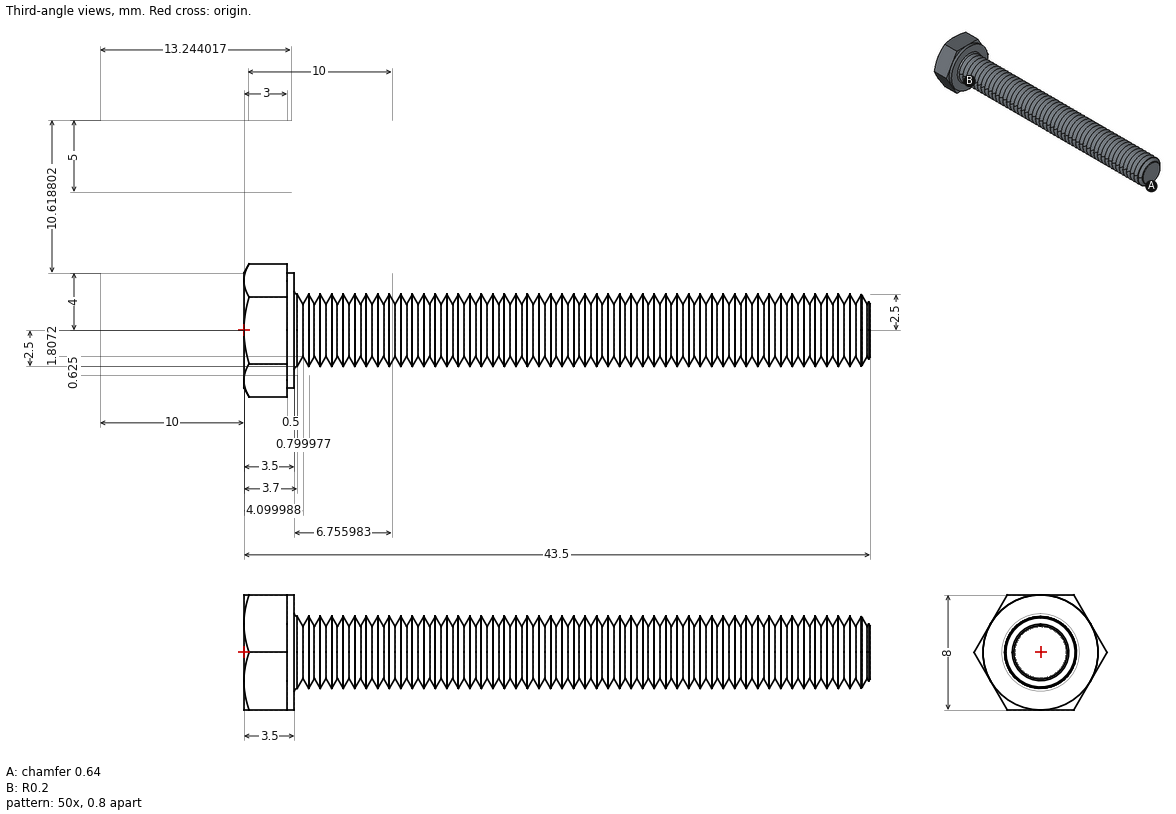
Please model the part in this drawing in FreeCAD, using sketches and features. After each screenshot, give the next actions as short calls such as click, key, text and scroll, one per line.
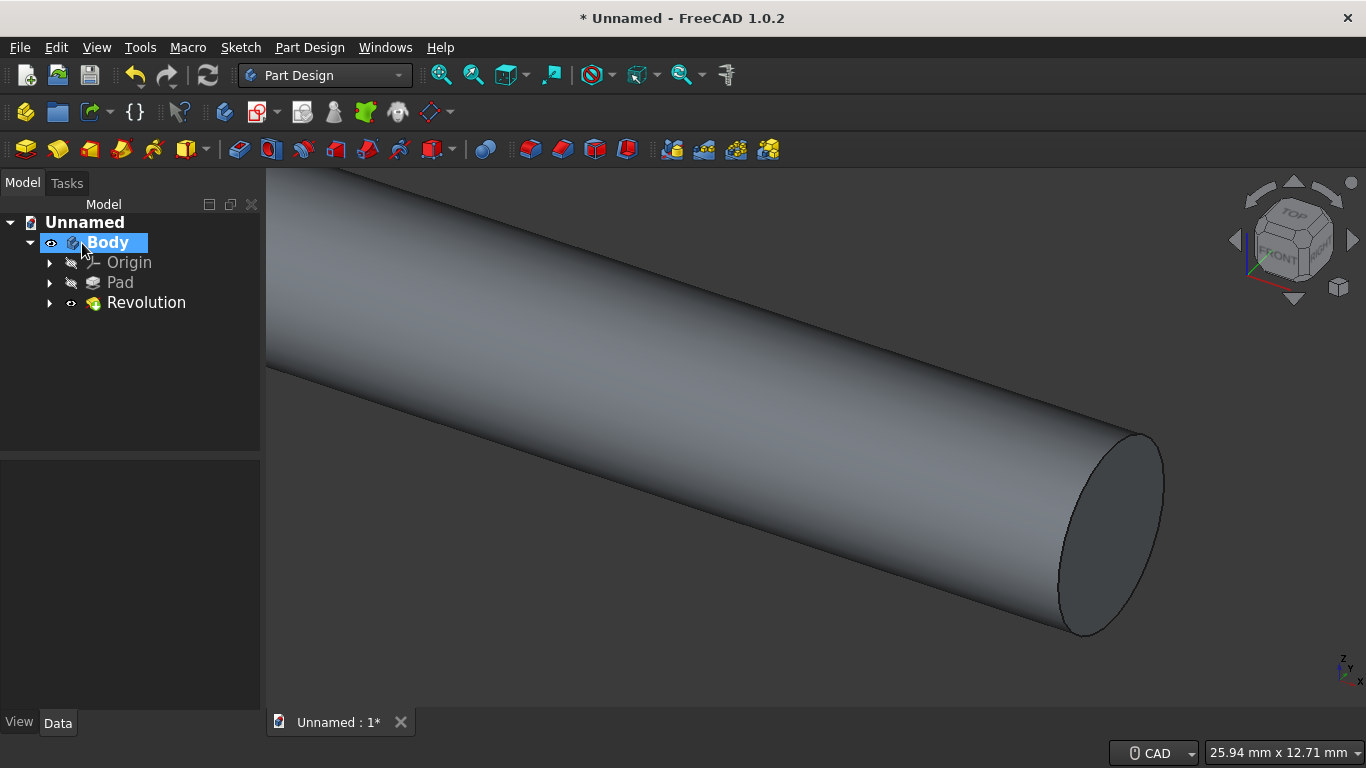
click(442, 76)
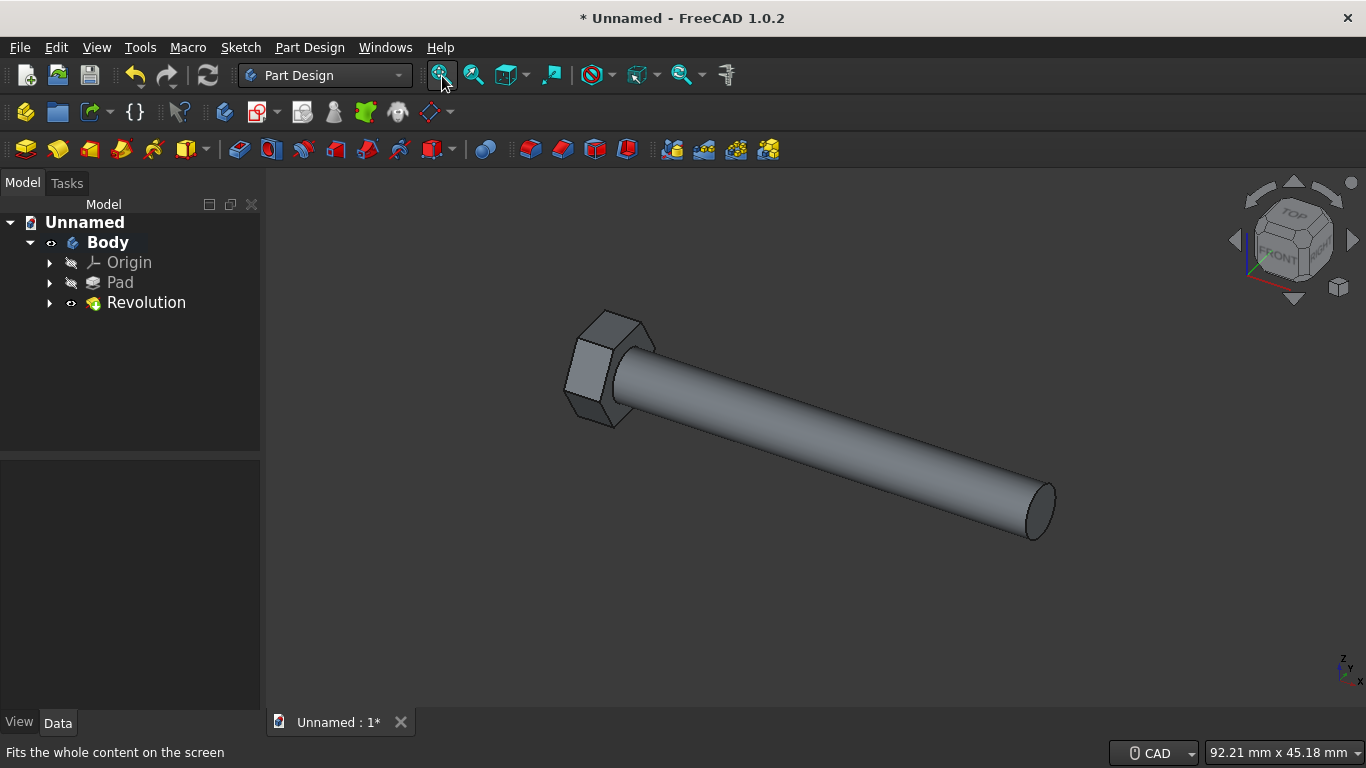
click(258, 112)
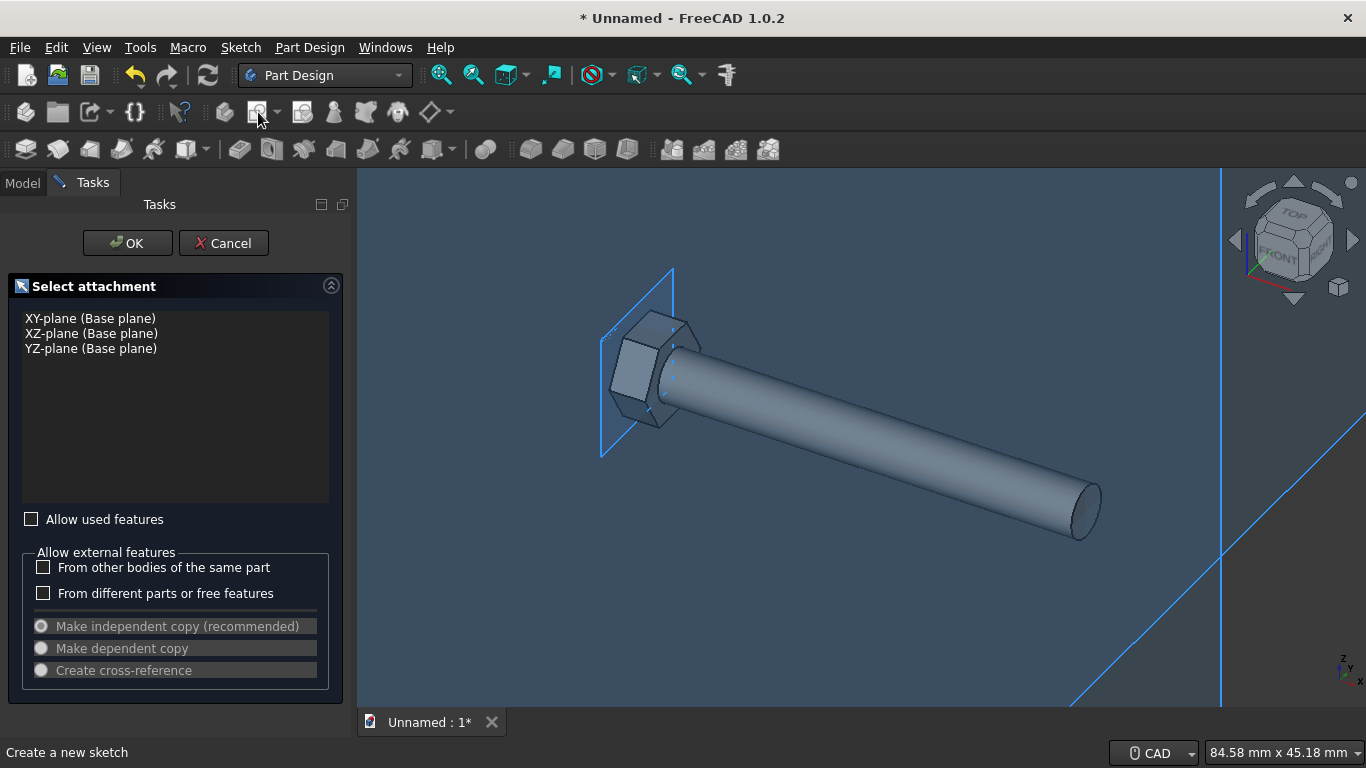
click(82, 318)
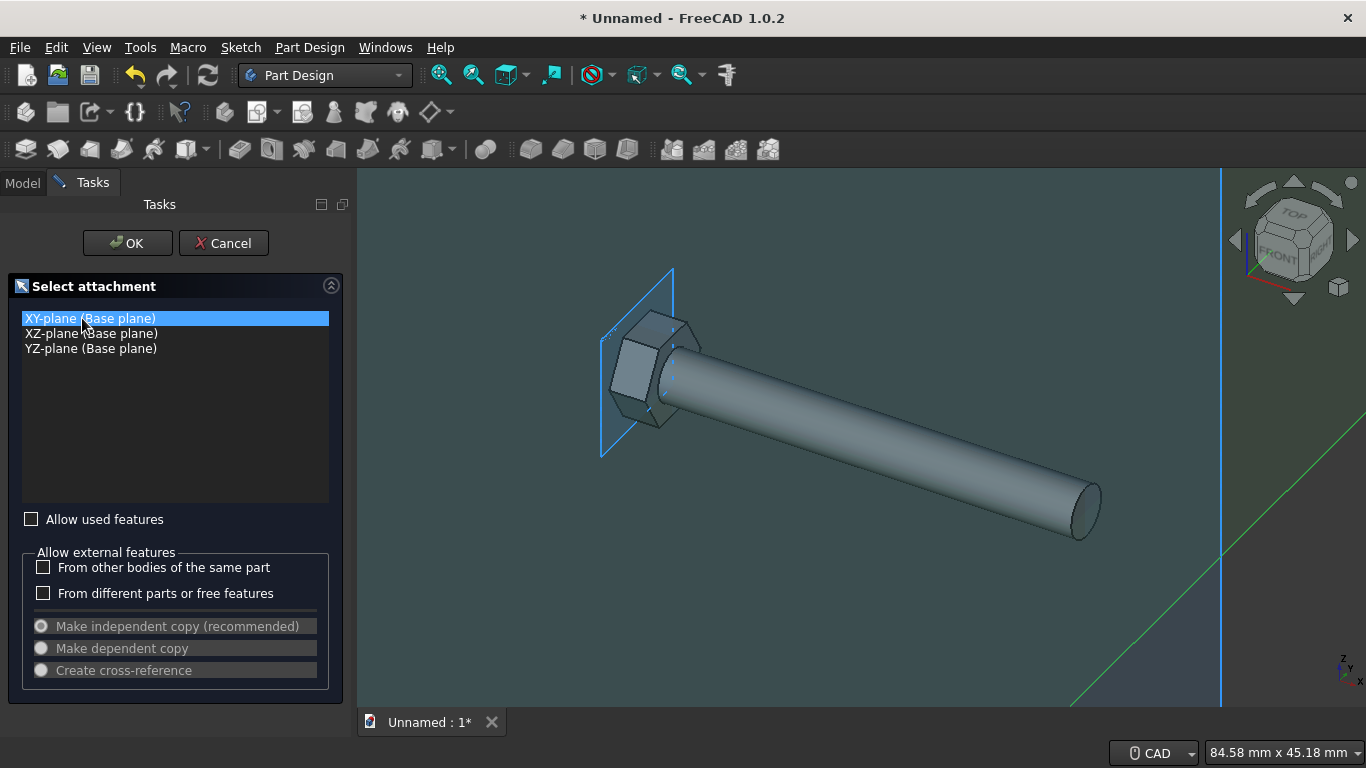
click(128, 243)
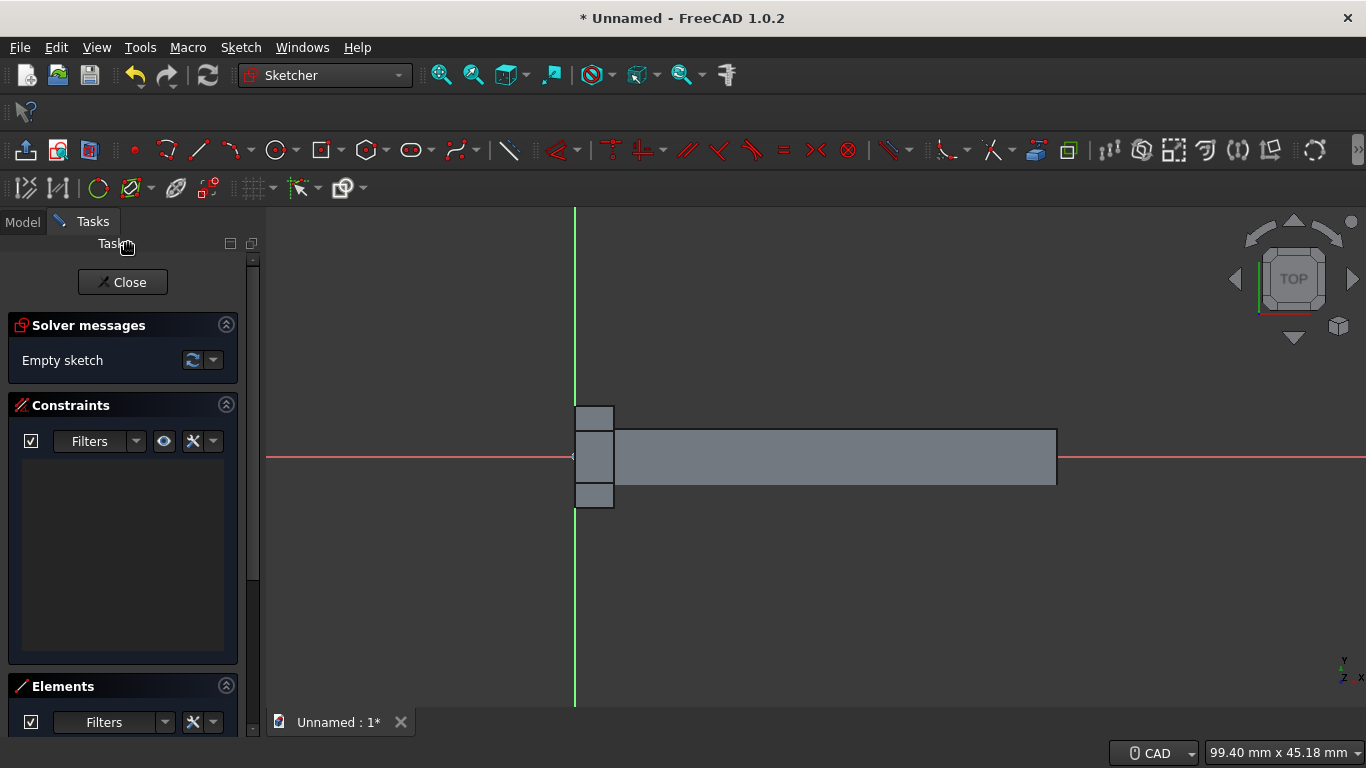
click(90, 150)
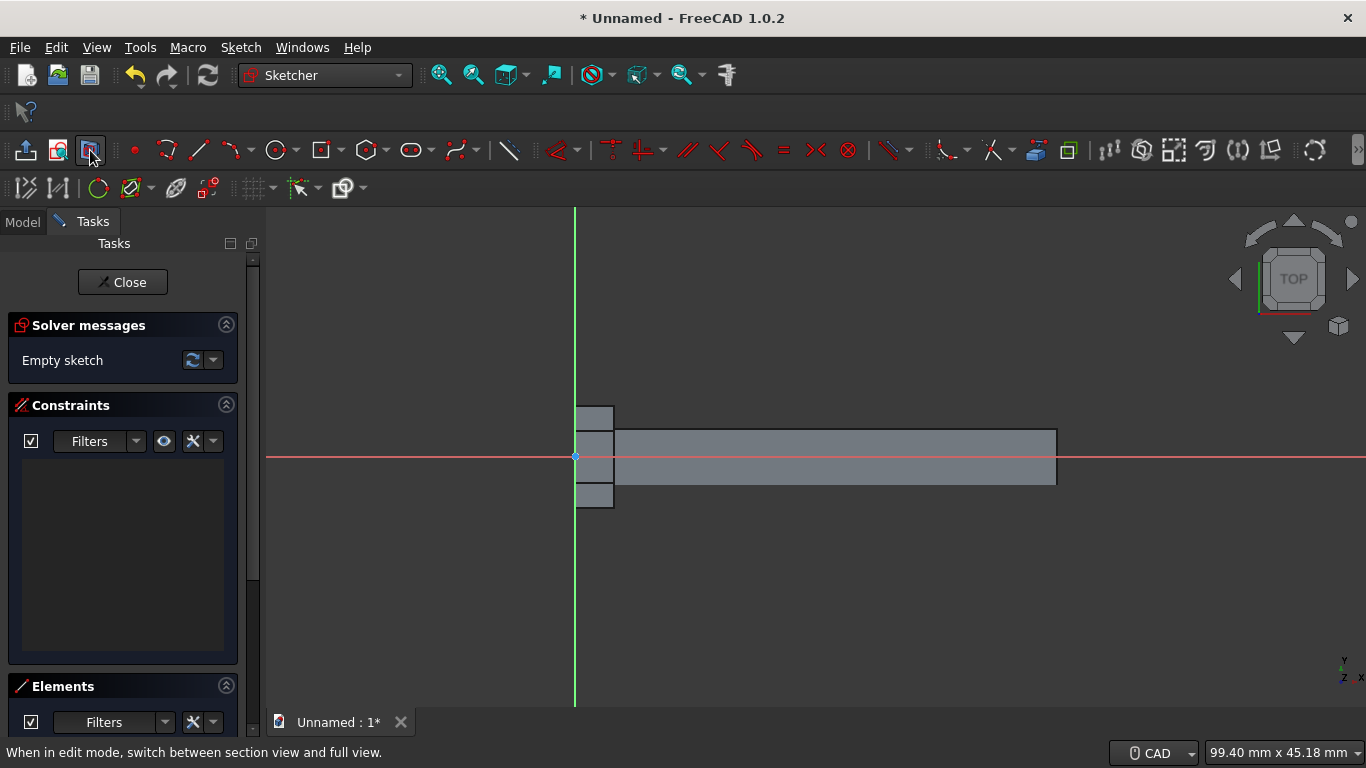
scroll(294, 278, up, 3)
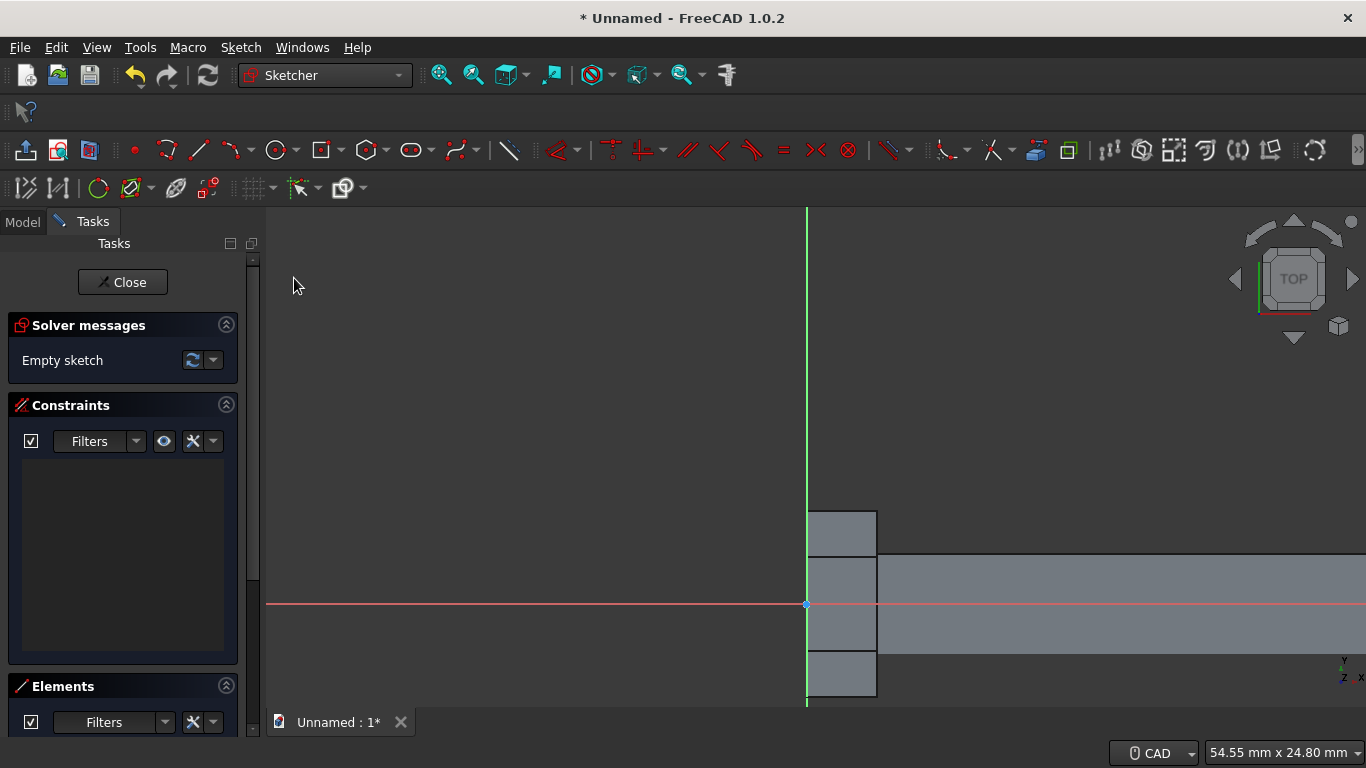
click(168, 150)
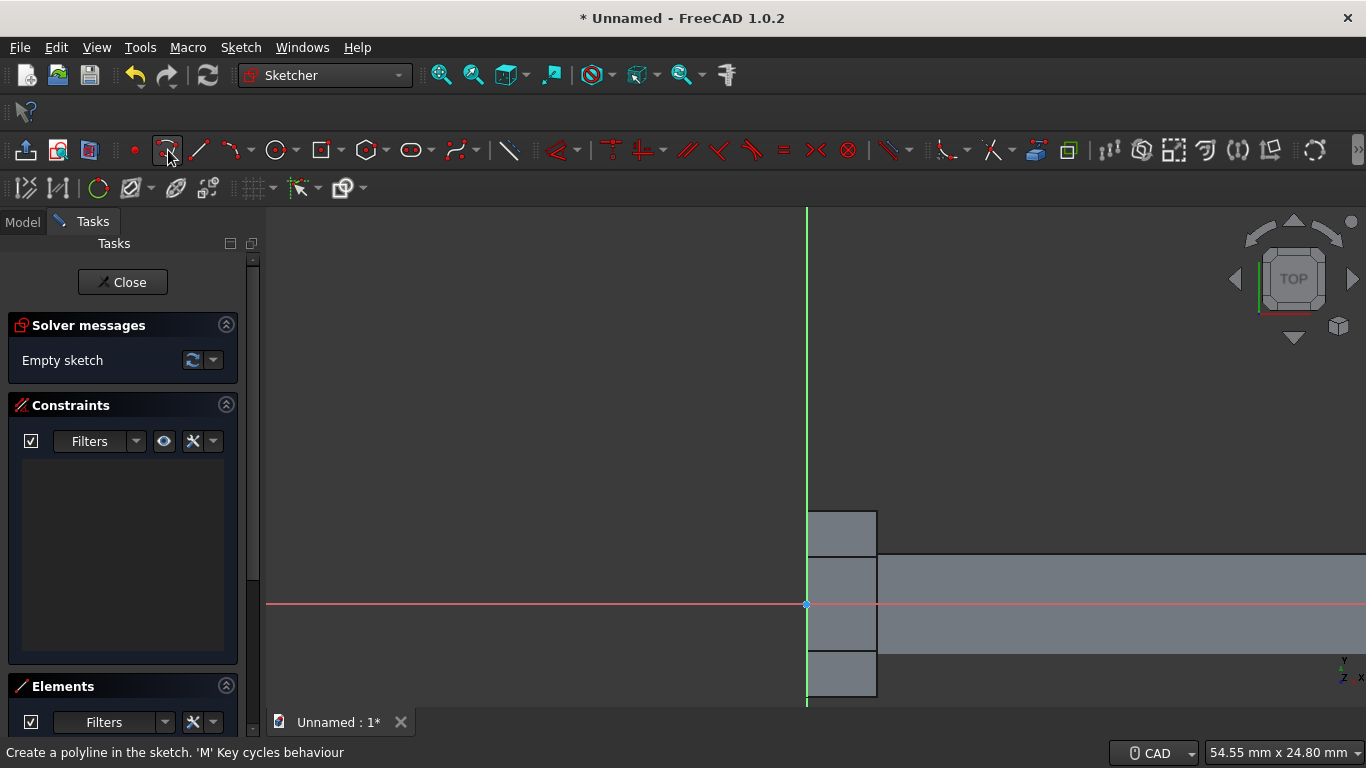
click(807, 523)
click(872, 410)
click(872, 309)
click(605, 309)
click(605, 523)
click(807, 524)
key(Escape)
key(Escape)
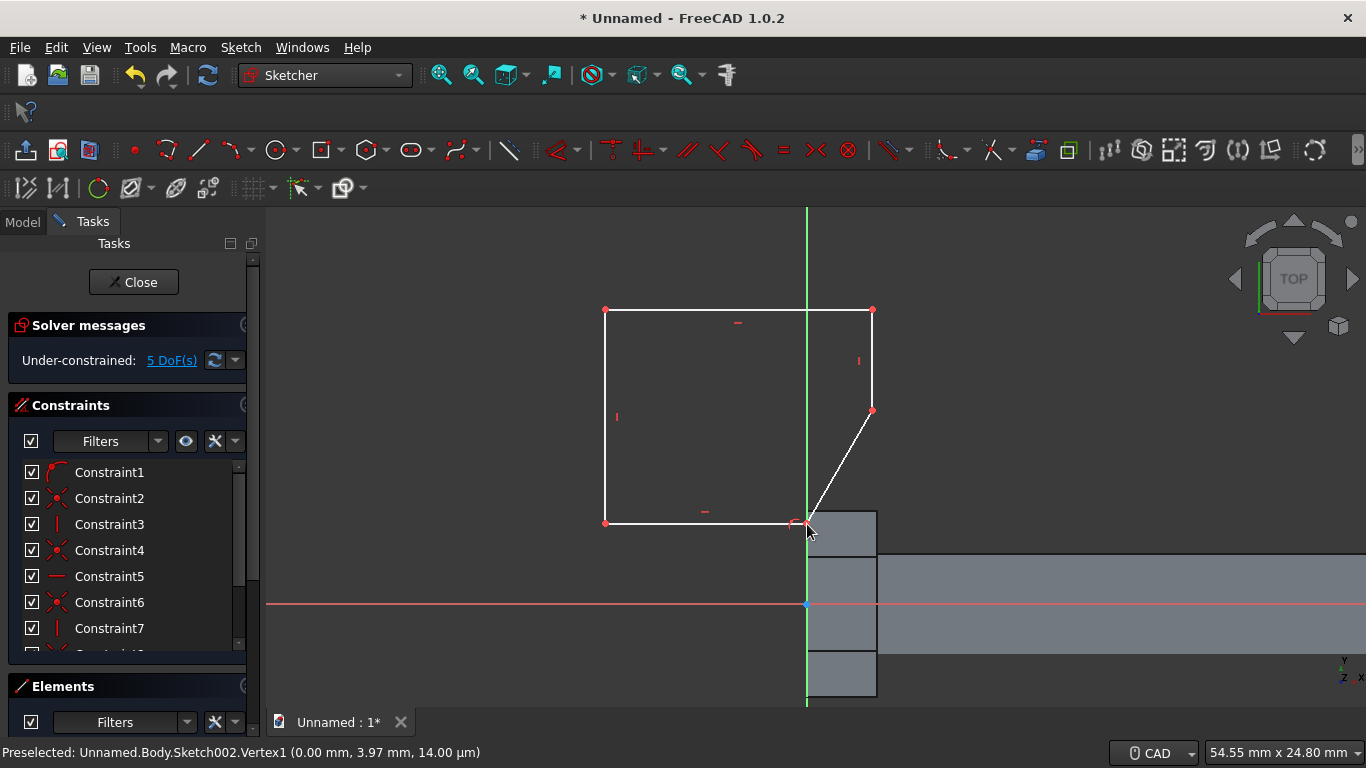
click(556, 150)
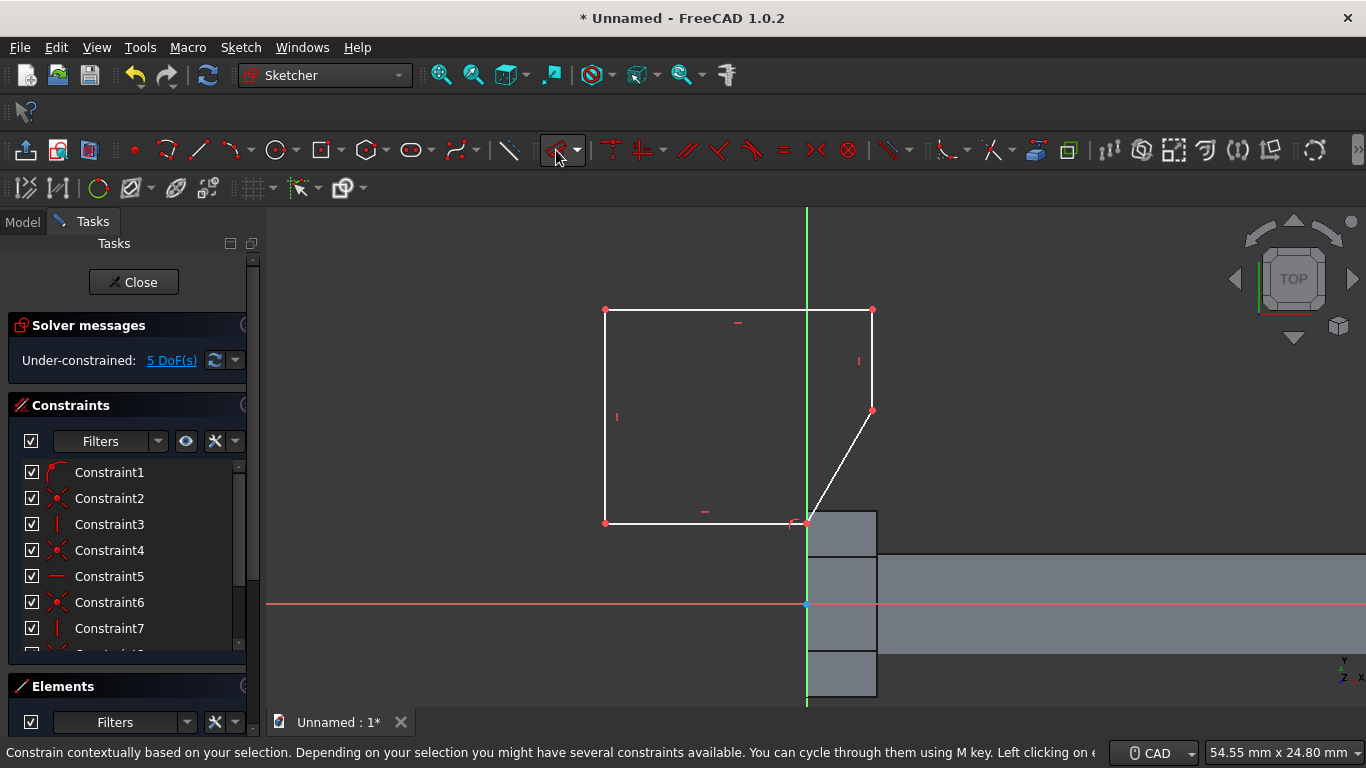
click(872, 381)
click(906, 360)